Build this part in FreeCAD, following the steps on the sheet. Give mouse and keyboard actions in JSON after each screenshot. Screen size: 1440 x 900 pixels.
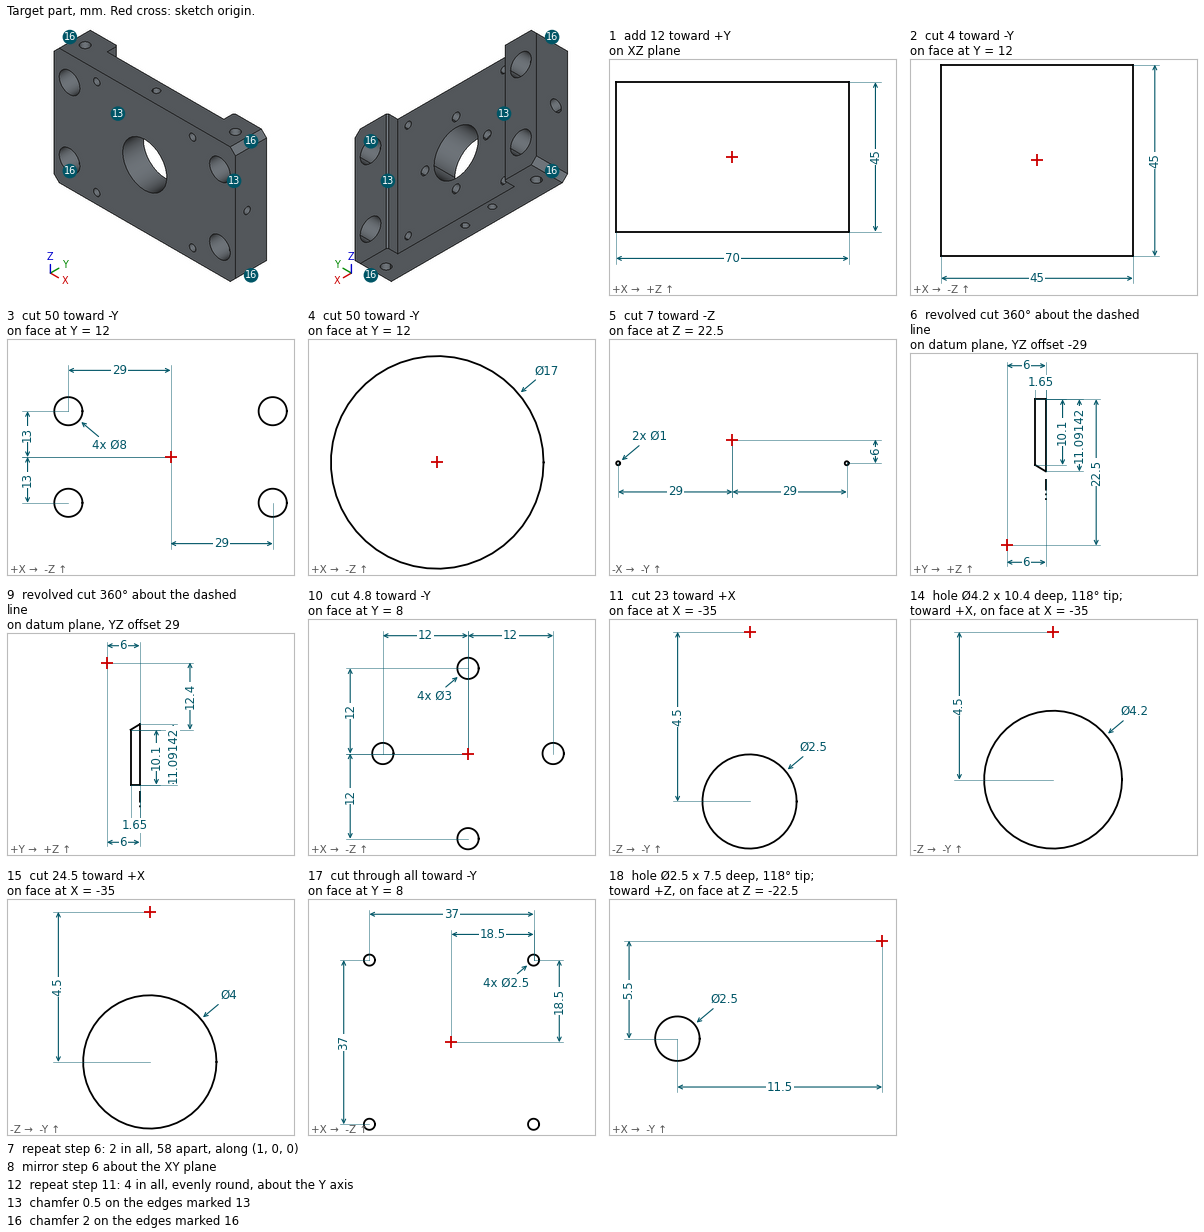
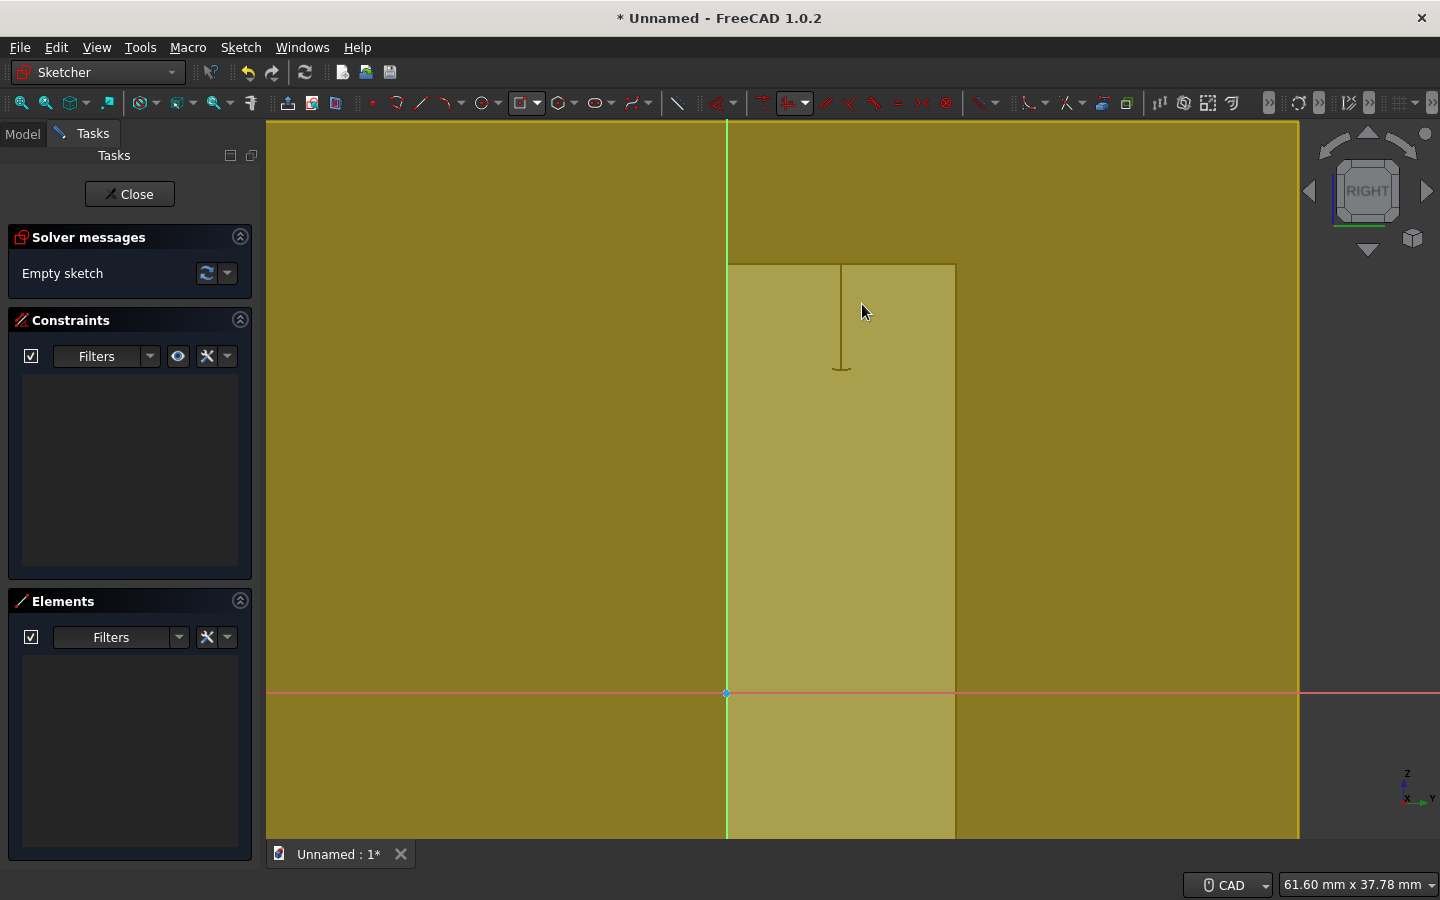
{"action": "left_click", "coordinate": [398, 104]}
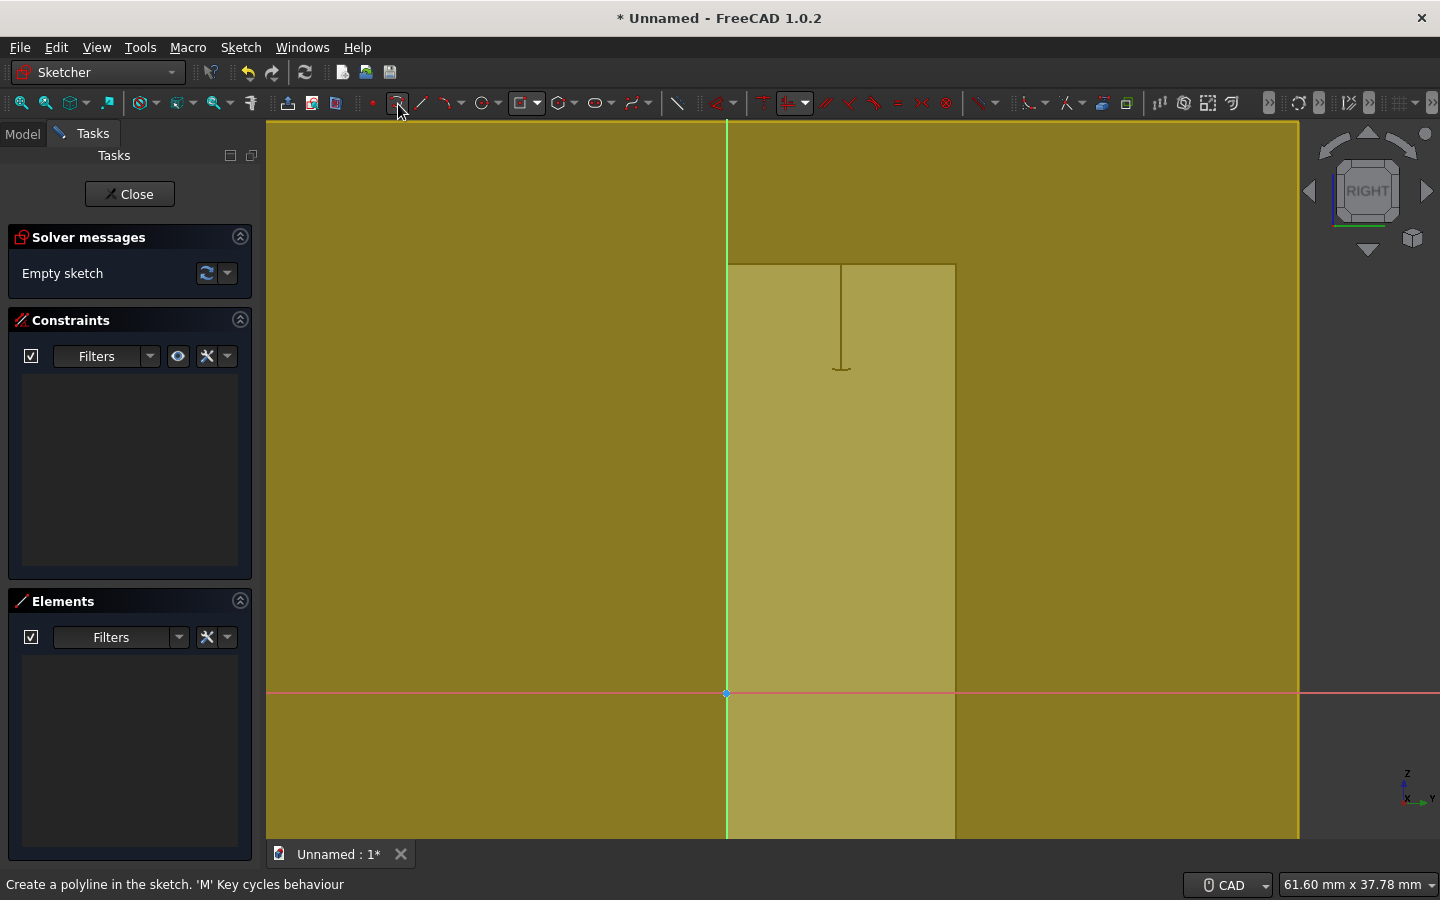
{"action": "left_click", "coordinate": [841, 476]}
{"action": "left_click", "coordinate": [841, 264]}
{"action": "left_click", "coordinate": [810, 264]}
{"action": "left_click", "coordinate": [810, 457]}
{"action": "left_click", "coordinate": [841, 477]}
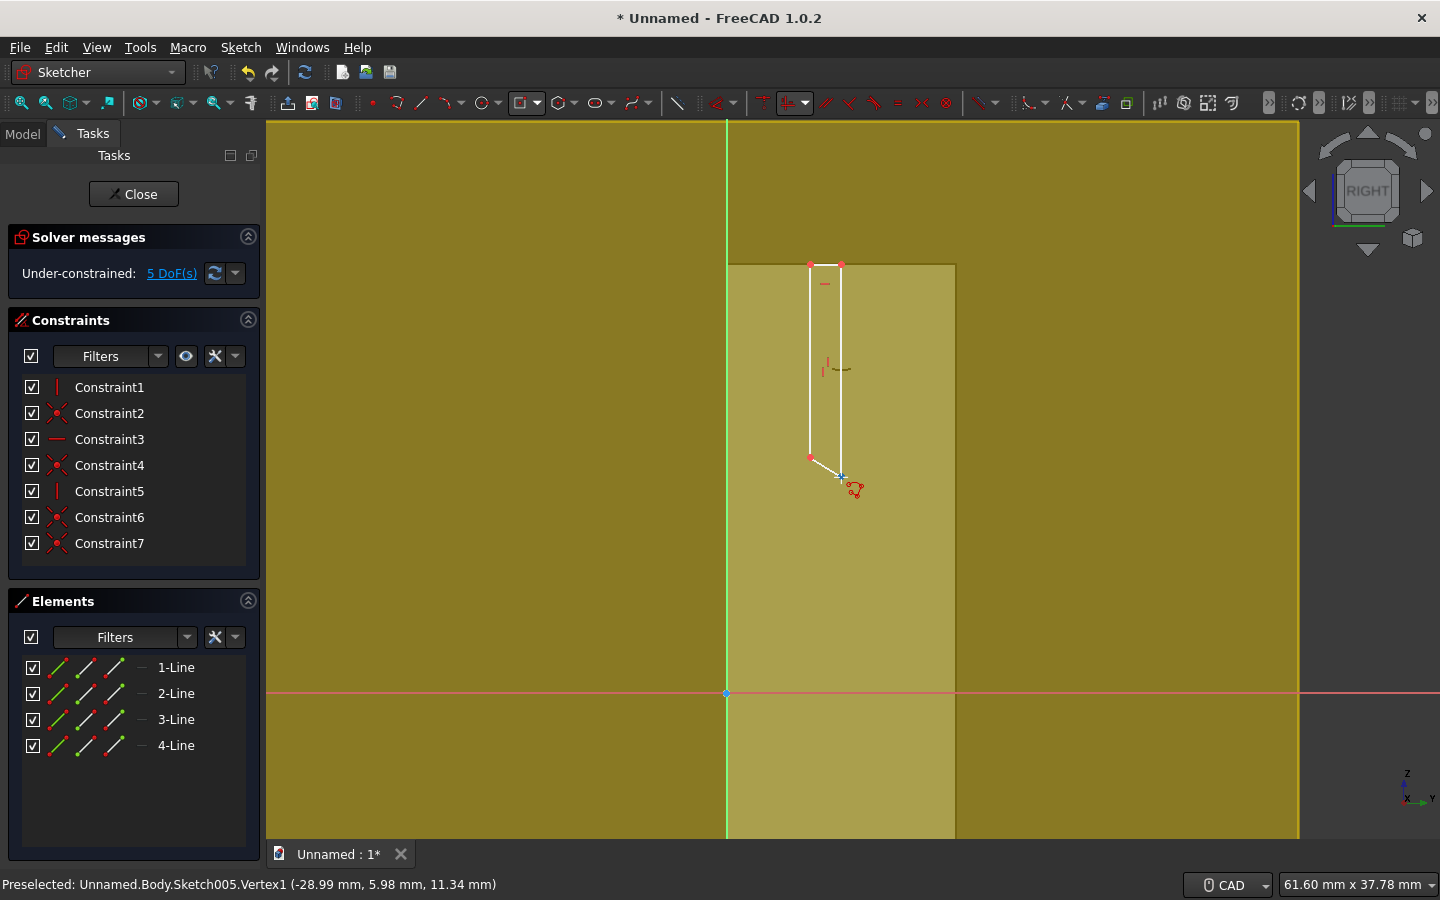
{"action": "left_click", "coordinate": [422, 104]}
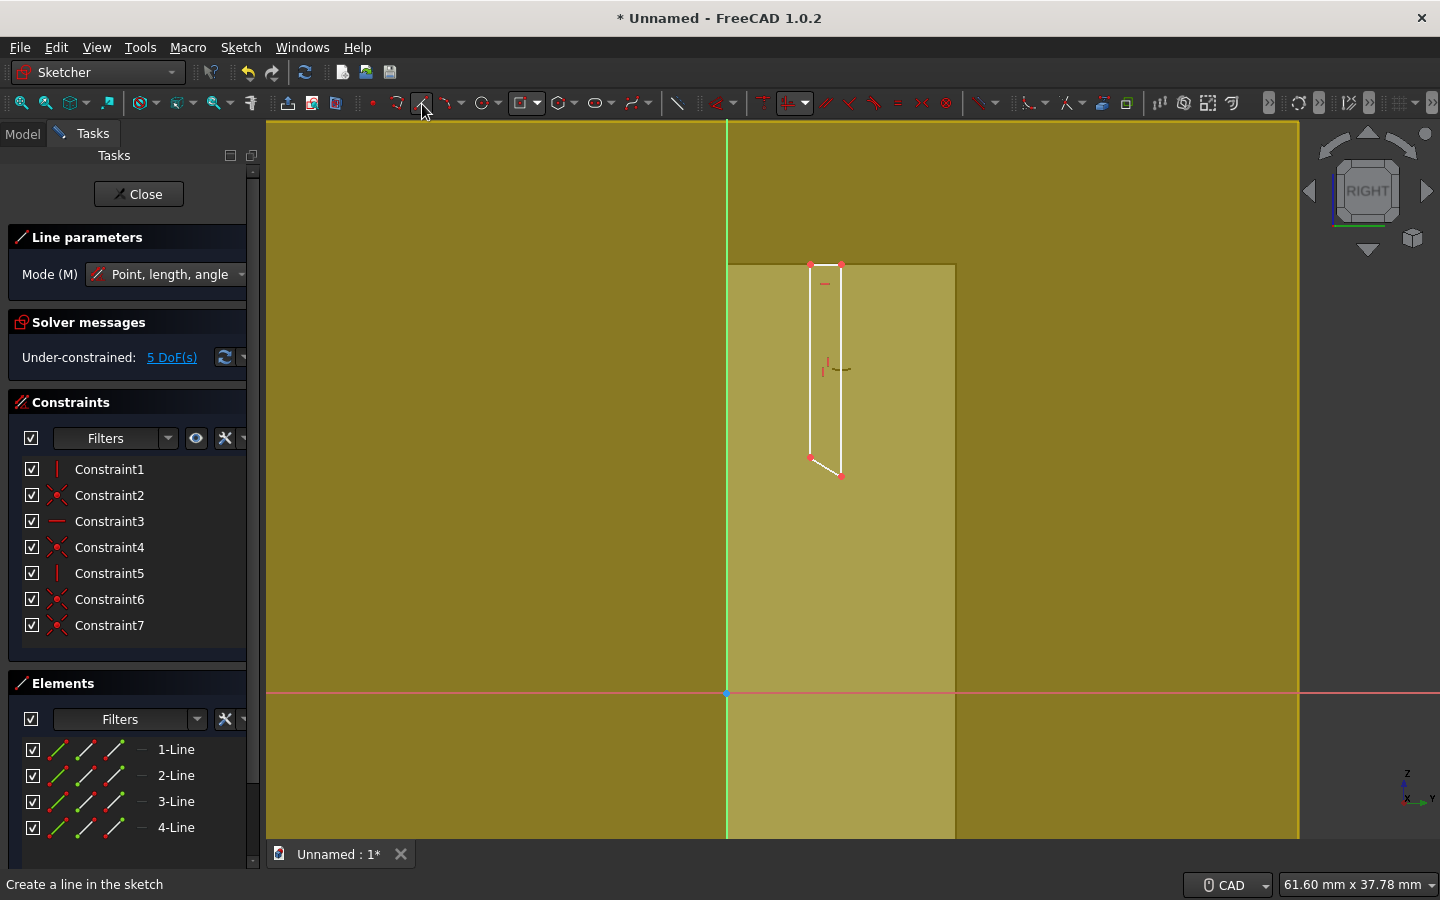
{"action": "left_click", "coordinate": [841, 497]}
{"action": "left_click", "coordinate": [841, 560]}
{"action": "key", "text": "Escape"}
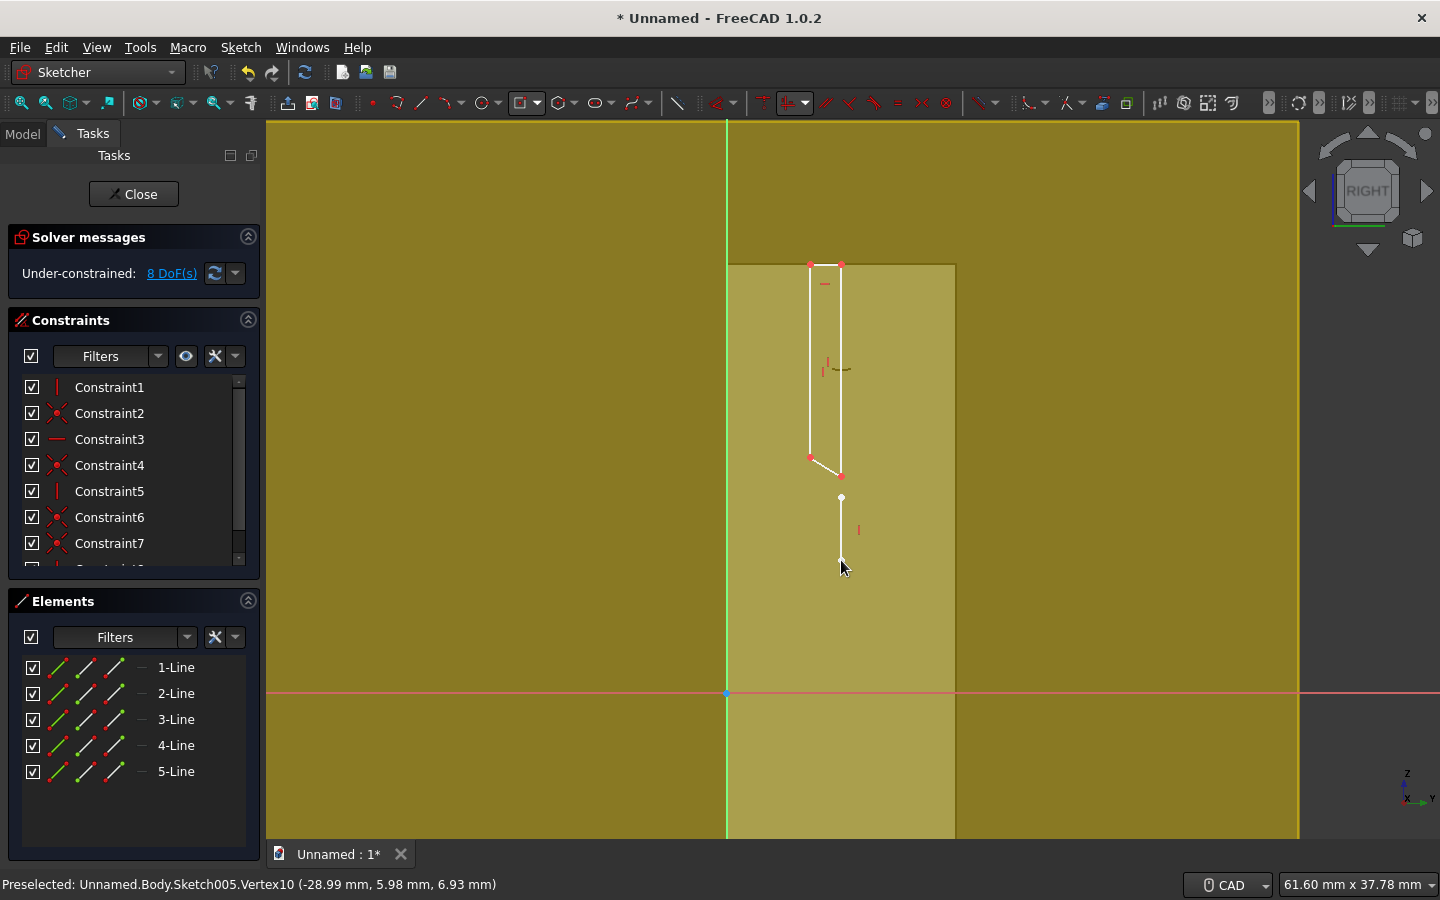
{"action": "left_click", "coordinate": [841, 517]}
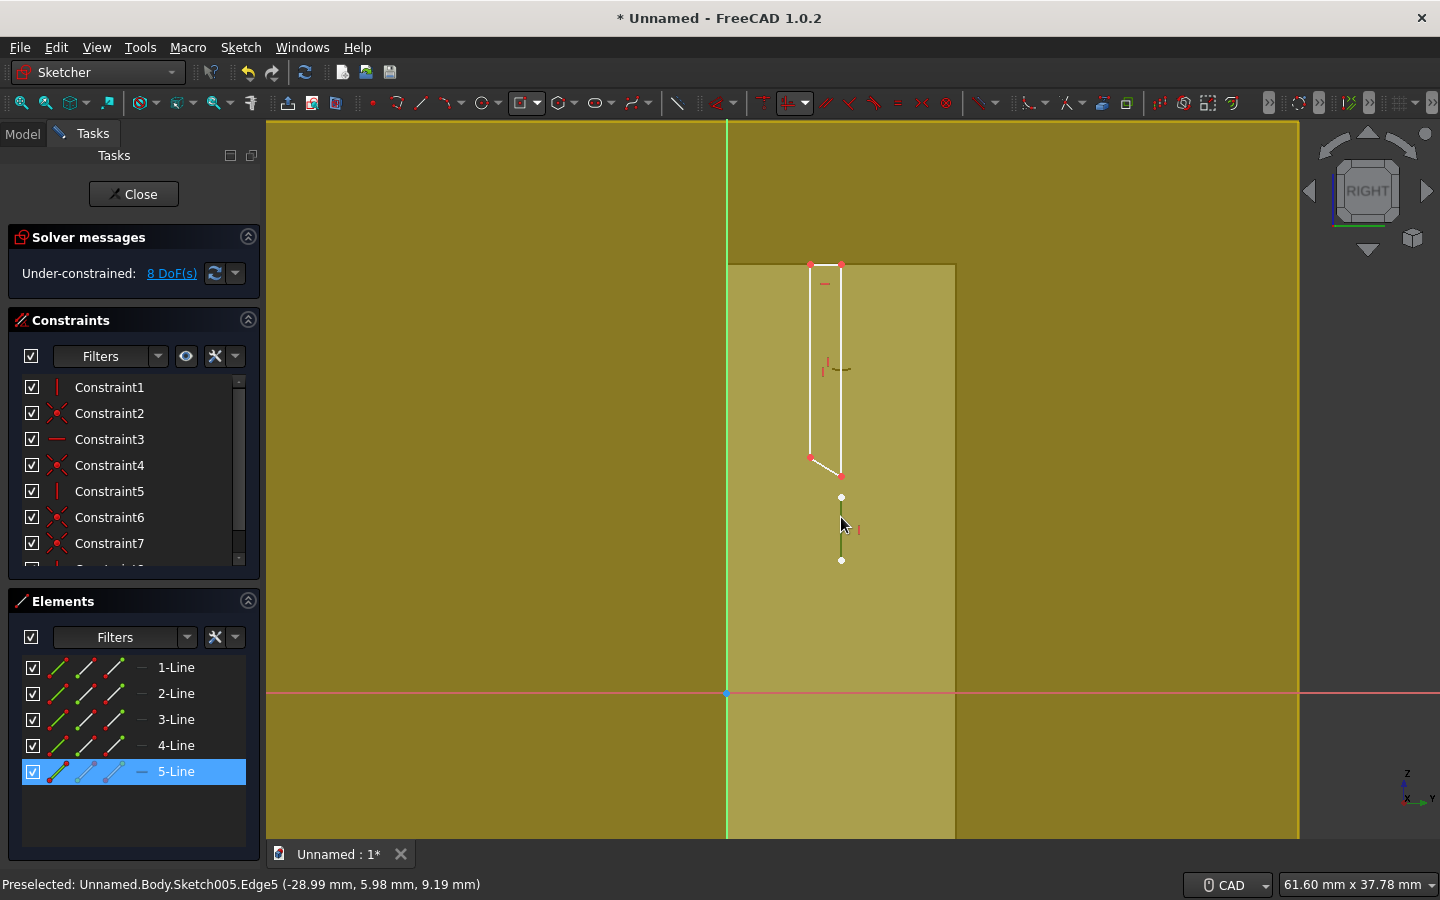
{"action": "left_click", "coordinate": [678, 104]}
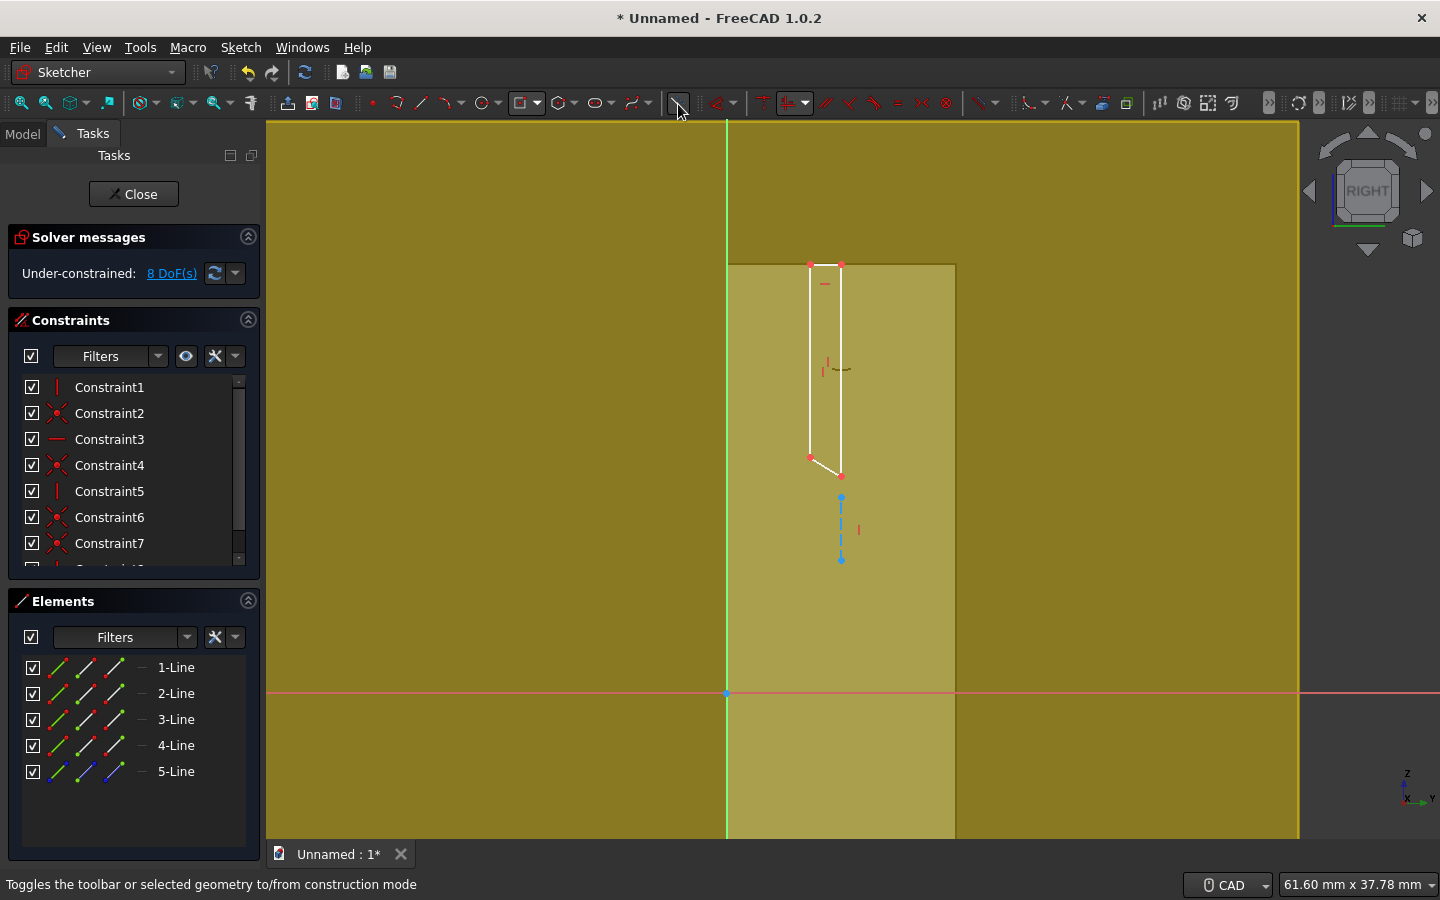
{"action": "left_click", "coordinate": [716, 104]}